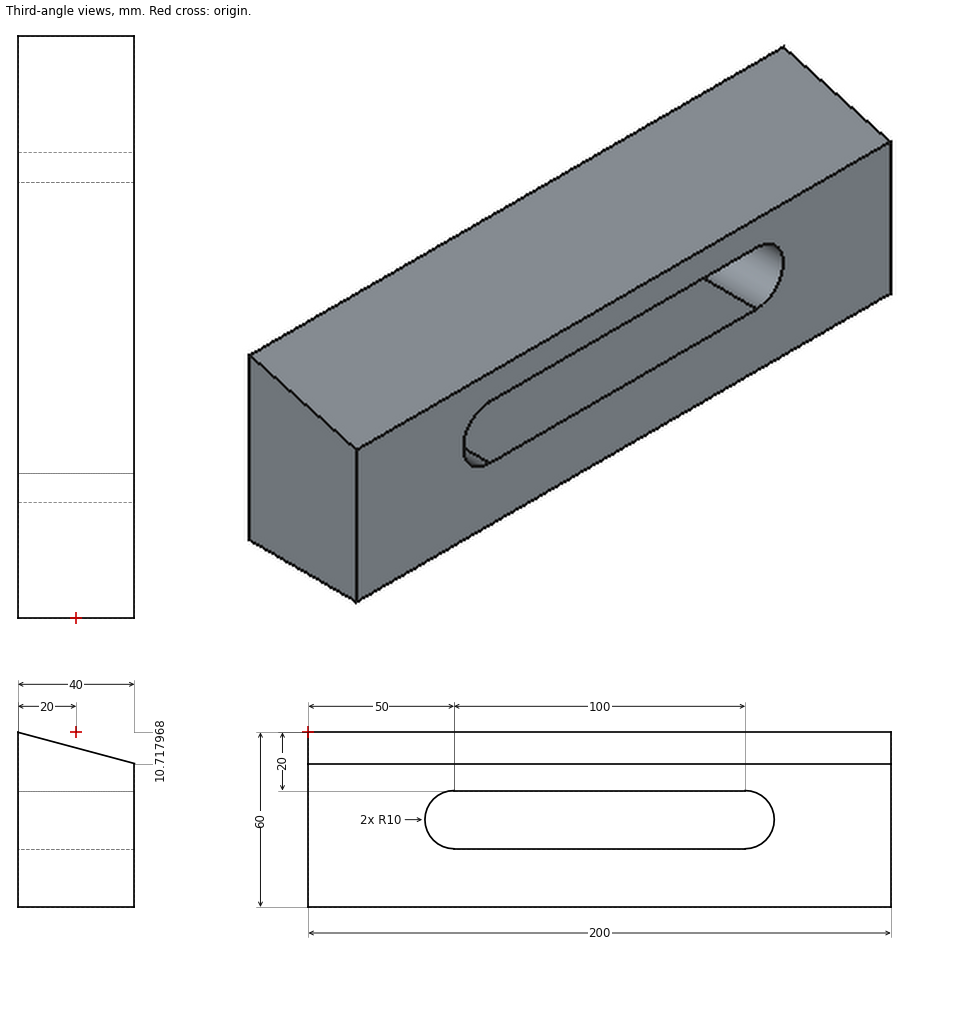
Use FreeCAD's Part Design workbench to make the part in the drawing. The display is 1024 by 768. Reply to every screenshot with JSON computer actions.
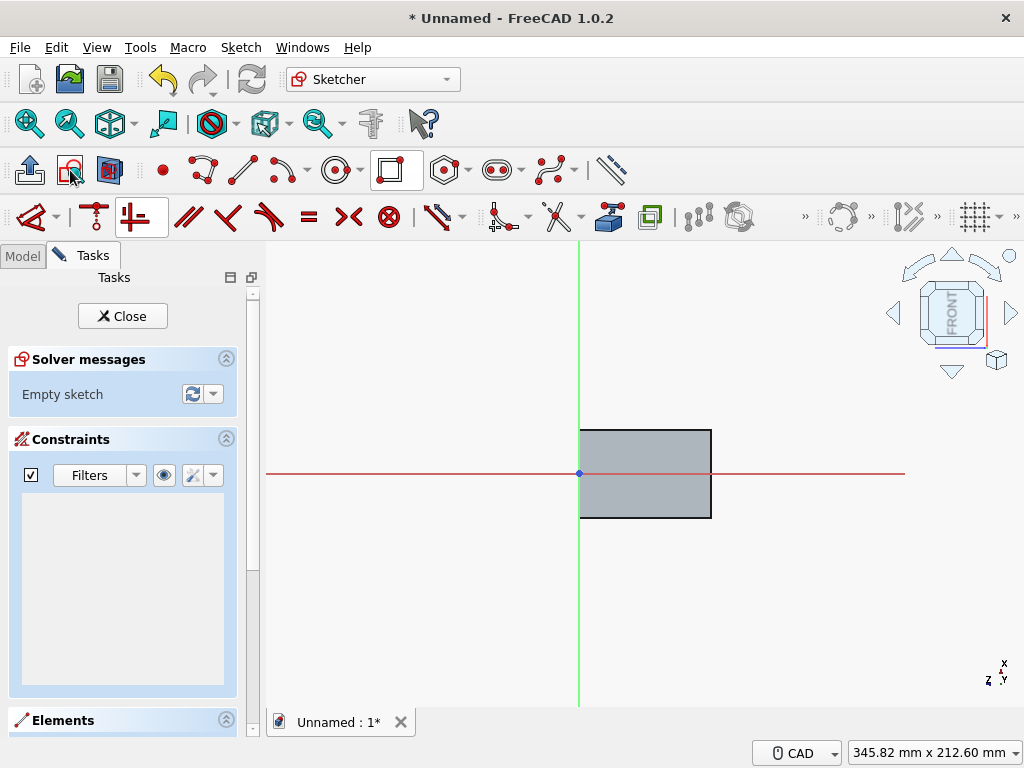
{"action": "scroll", "coordinate": [597, 474], "scroll_direction": "up", "scroll_amount": 6}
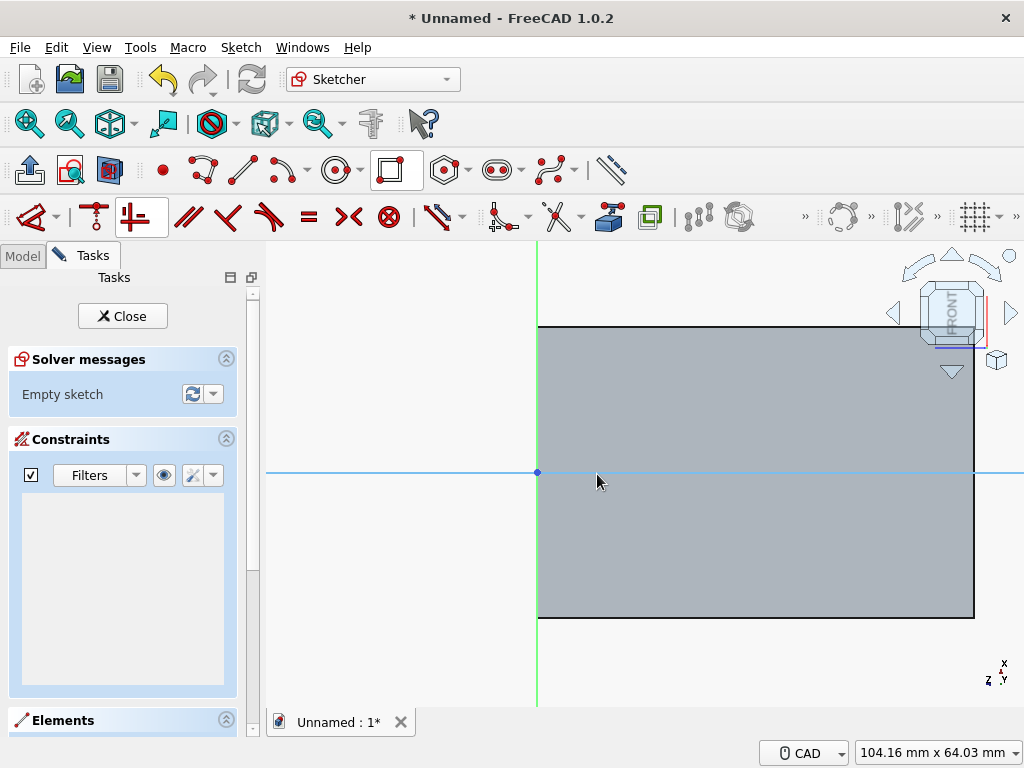
{"action": "left_click", "coordinate": [204, 170]}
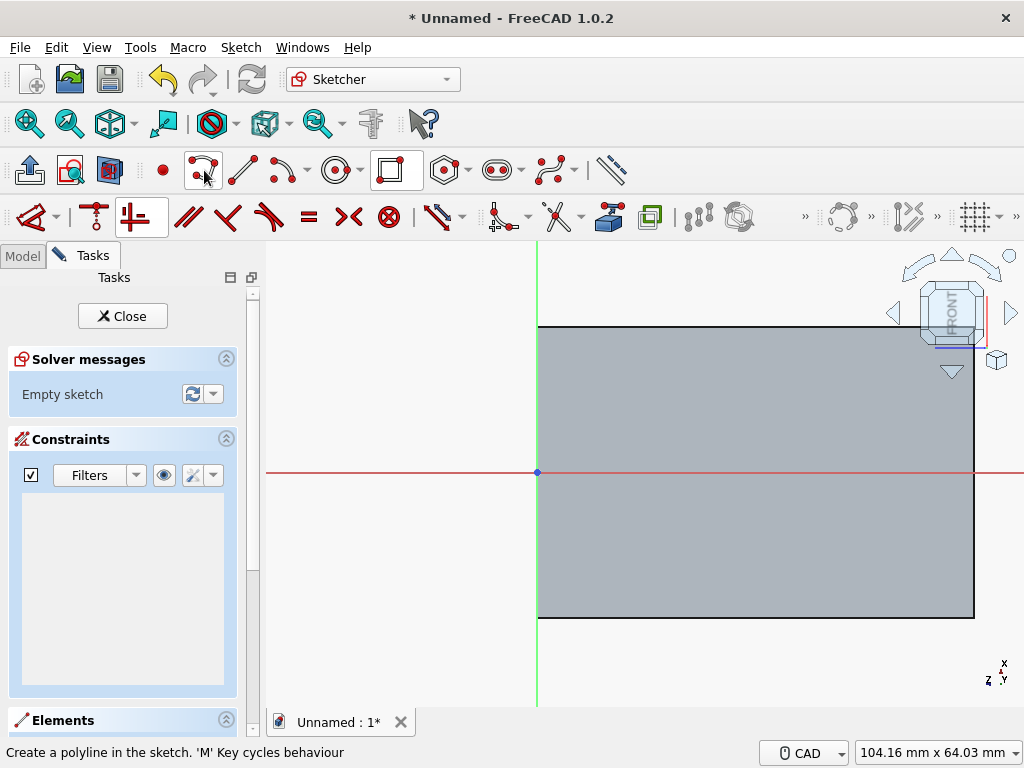
{"action": "left_click", "coordinate": [537, 618]}
{"action": "left_click", "coordinate": [615, 327]}
{"action": "left_click", "coordinate": [546, 327]}
{"action": "left_click", "coordinate": [537, 619]}
{"action": "key", "text": "Escape"}
{"action": "key", "text": "Escape"}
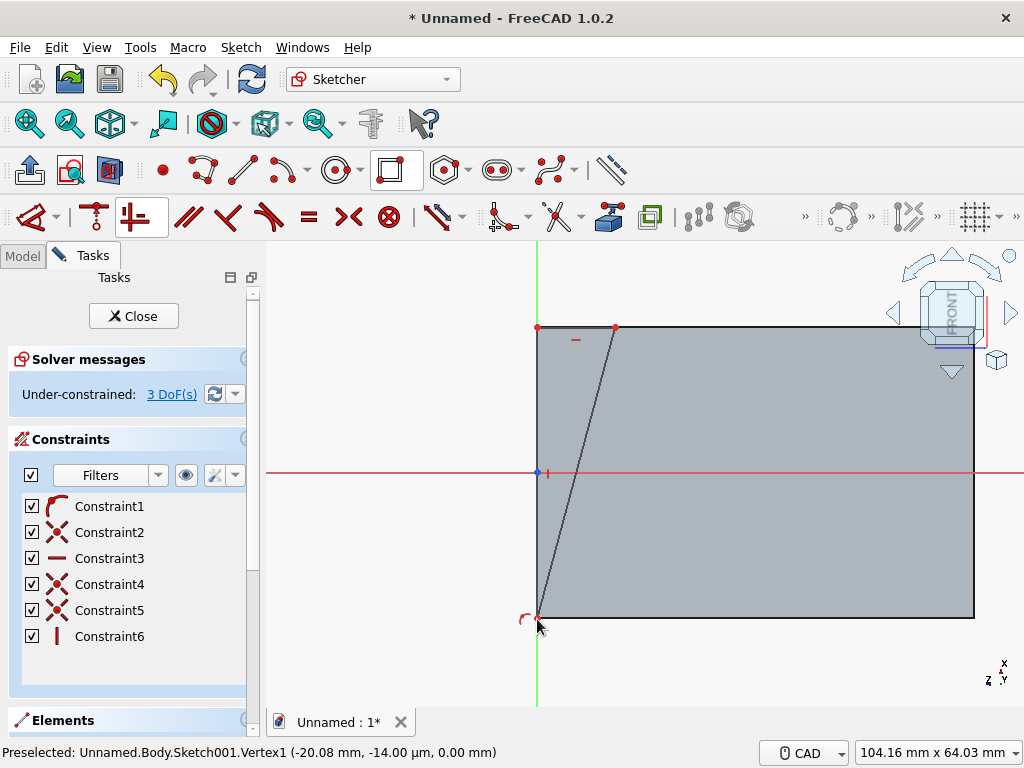
{"action": "left_click", "coordinate": [32, 218]}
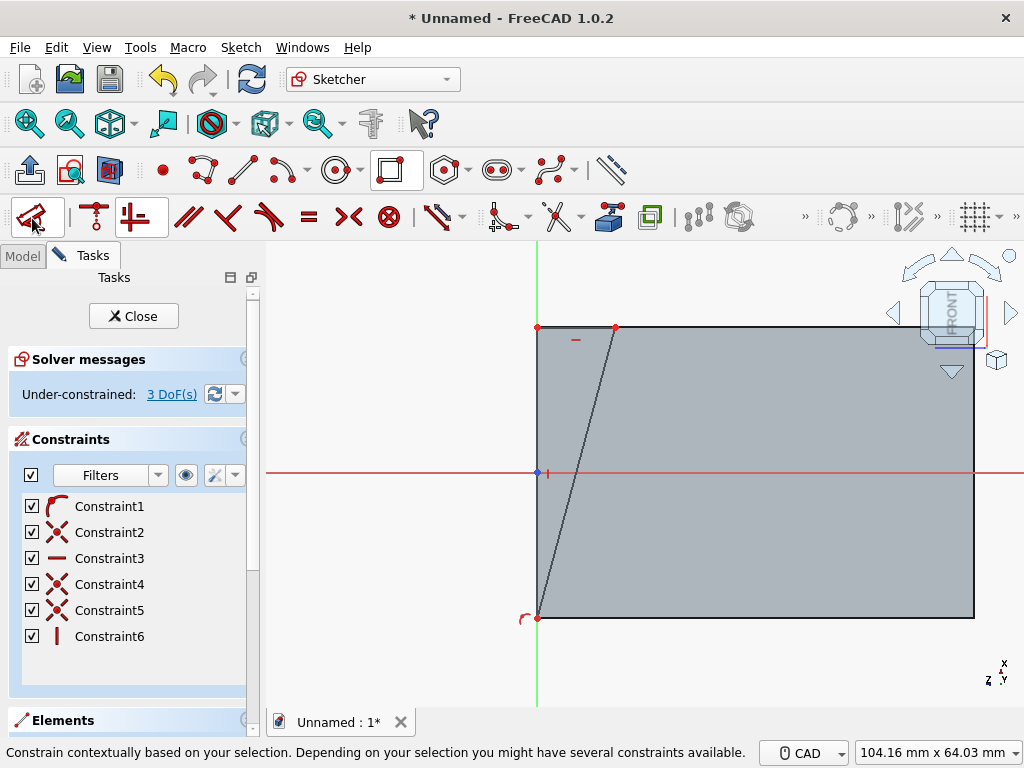
{"action": "left_click", "coordinate": [537, 415]}
{"action": "left_click", "coordinate": [503, 407]}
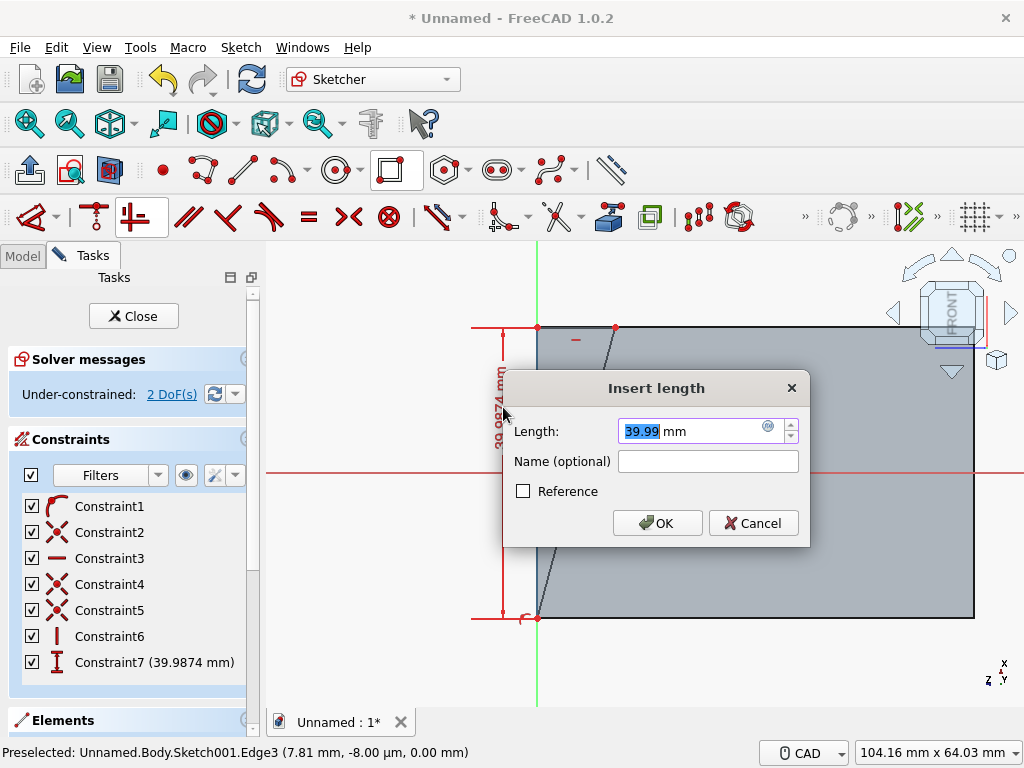
{"action": "type", "text": "40"}
{"action": "key", "text": "Return"}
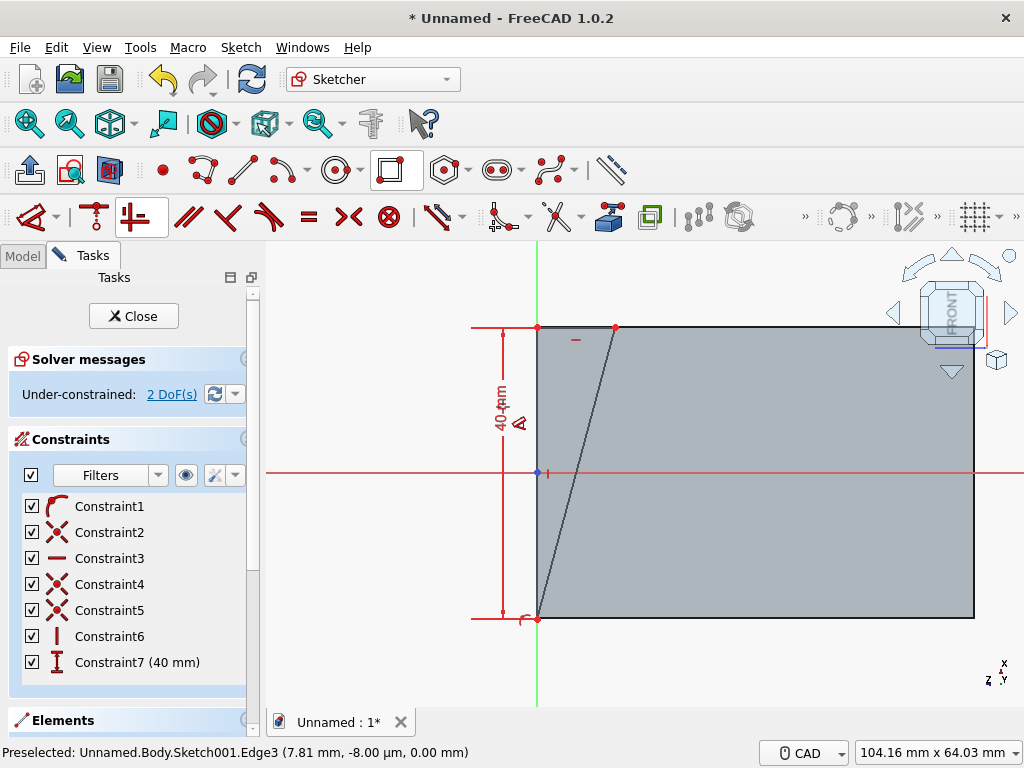
{"action": "left_click", "coordinate": [537, 619]}
{"action": "left_click", "coordinate": [503, 546]}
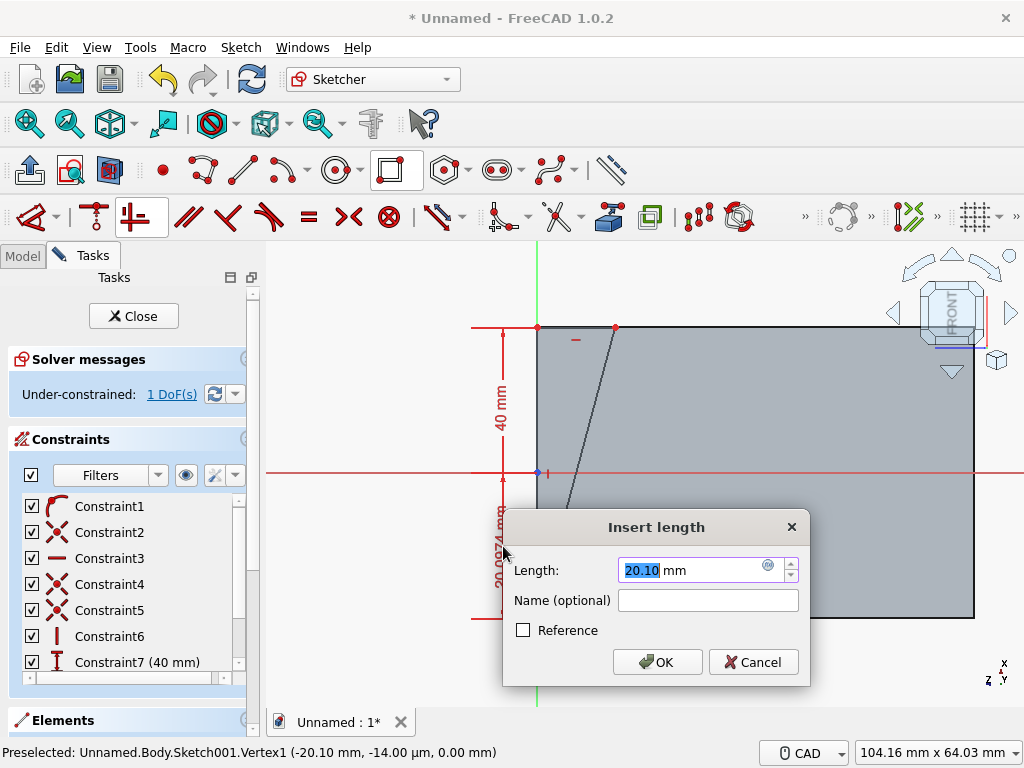
{"action": "type", "text": "20"}
{"action": "key", "text": "Return"}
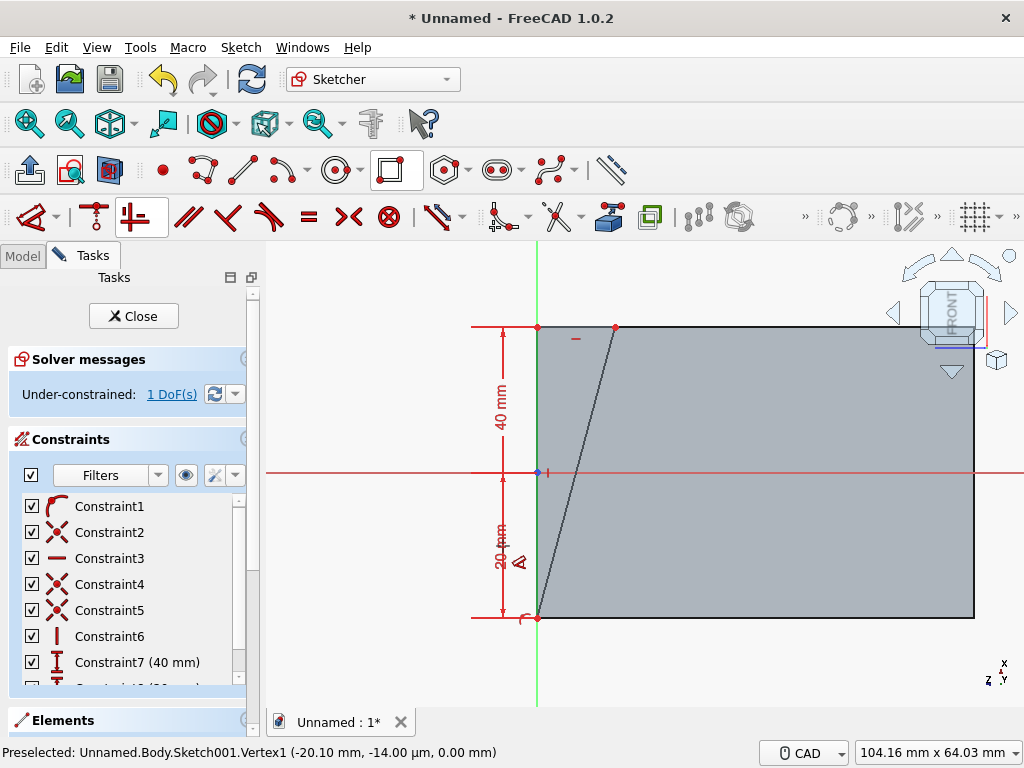
{"action": "left_click", "coordinate": [592, 327]}
{"action": "left_click", "coordinate": [576, 293]}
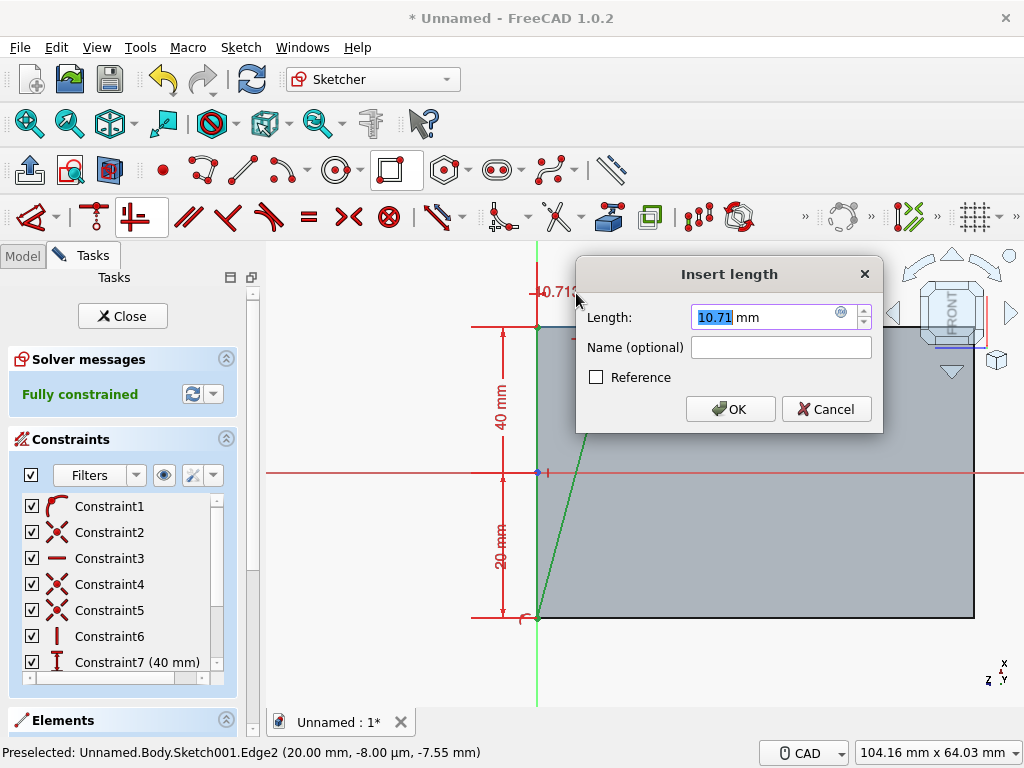
{"action": "type", "text": "10.717968"}
{"action": "key", "text": "Return"}
{"action": "key", "text": "Escape"}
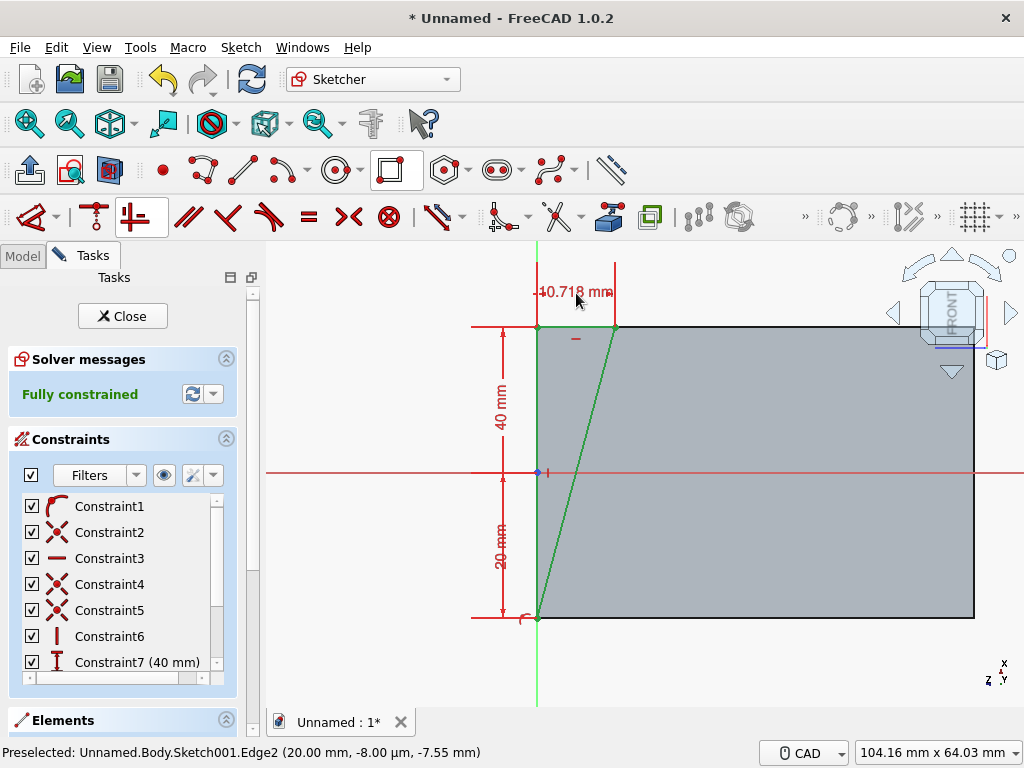
{"action": "left_click", "coordinate": [123, 316]}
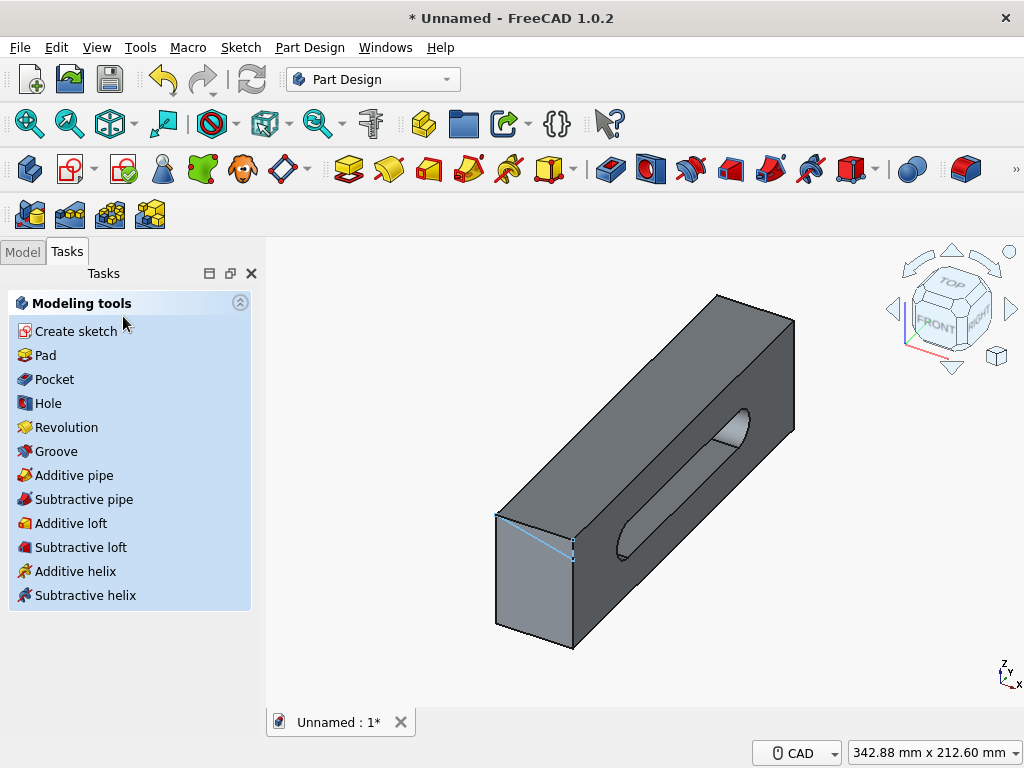
{"action": "left_click", "coordinate": [612, 170]}